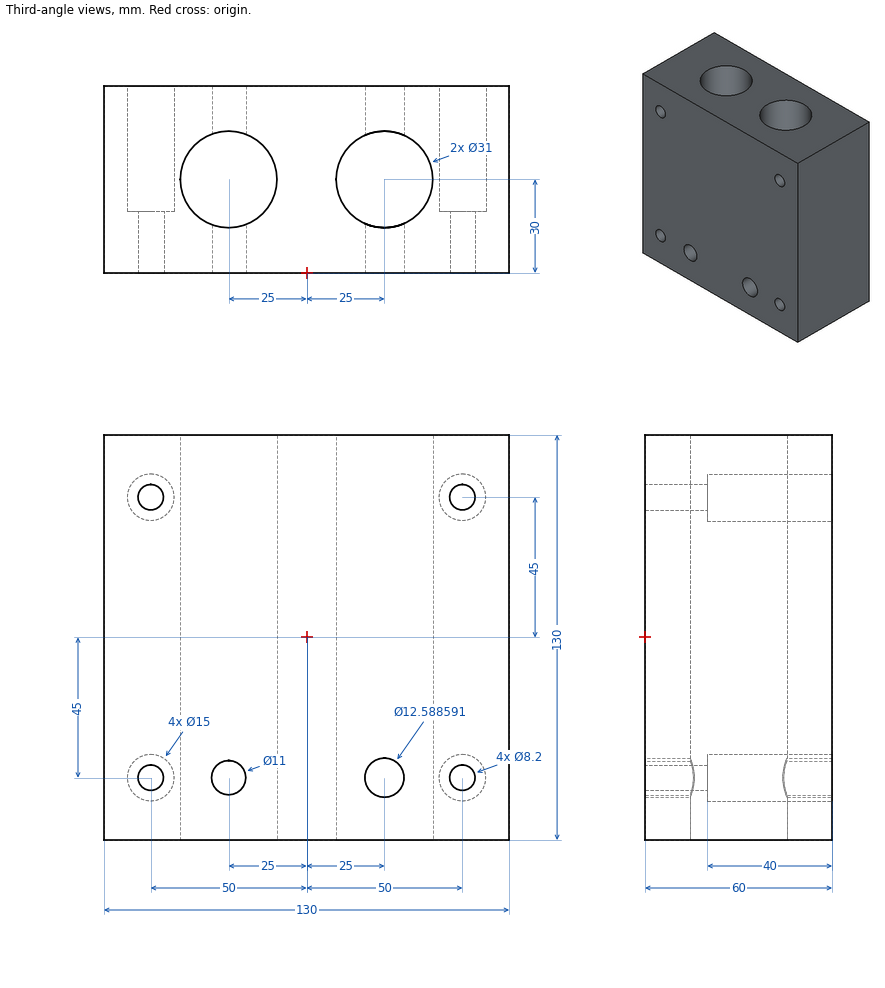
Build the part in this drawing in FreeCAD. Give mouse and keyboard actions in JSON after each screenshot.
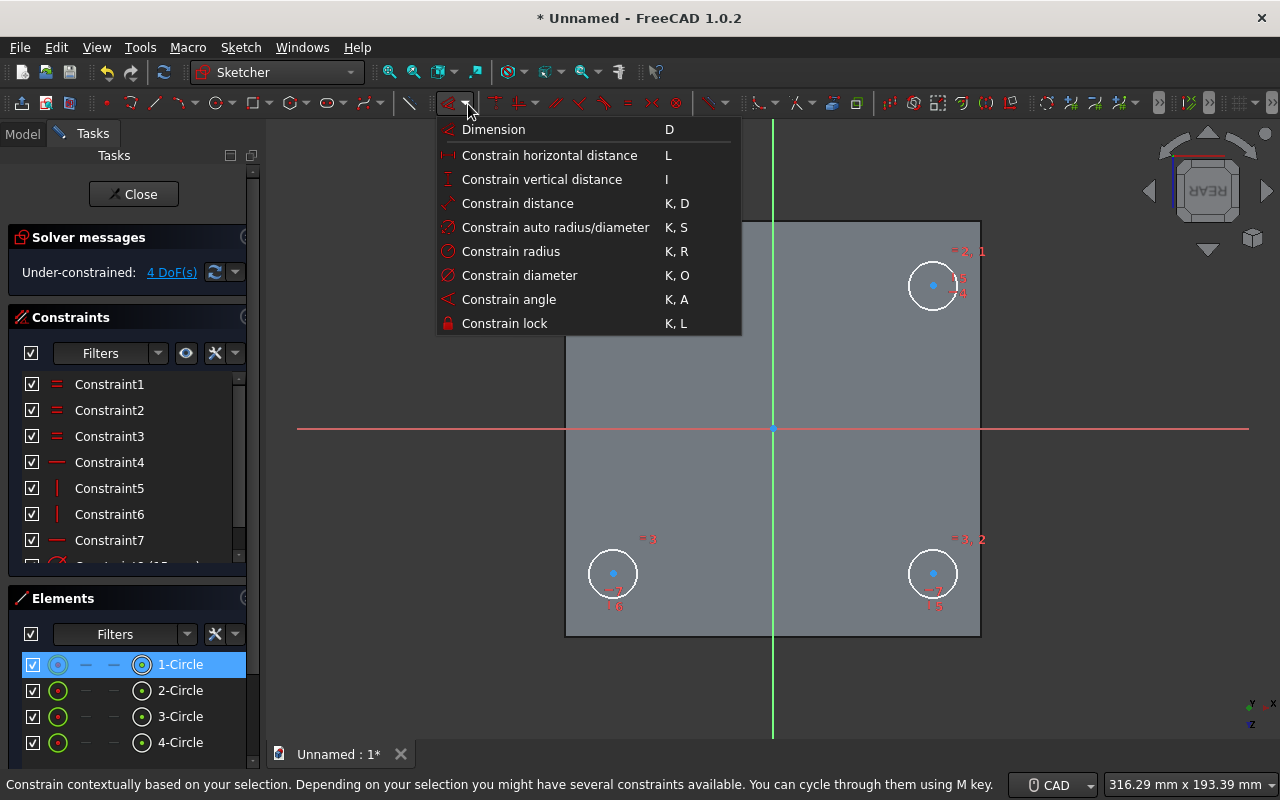
{"action": "left_click", "coordinate": [589, 155]}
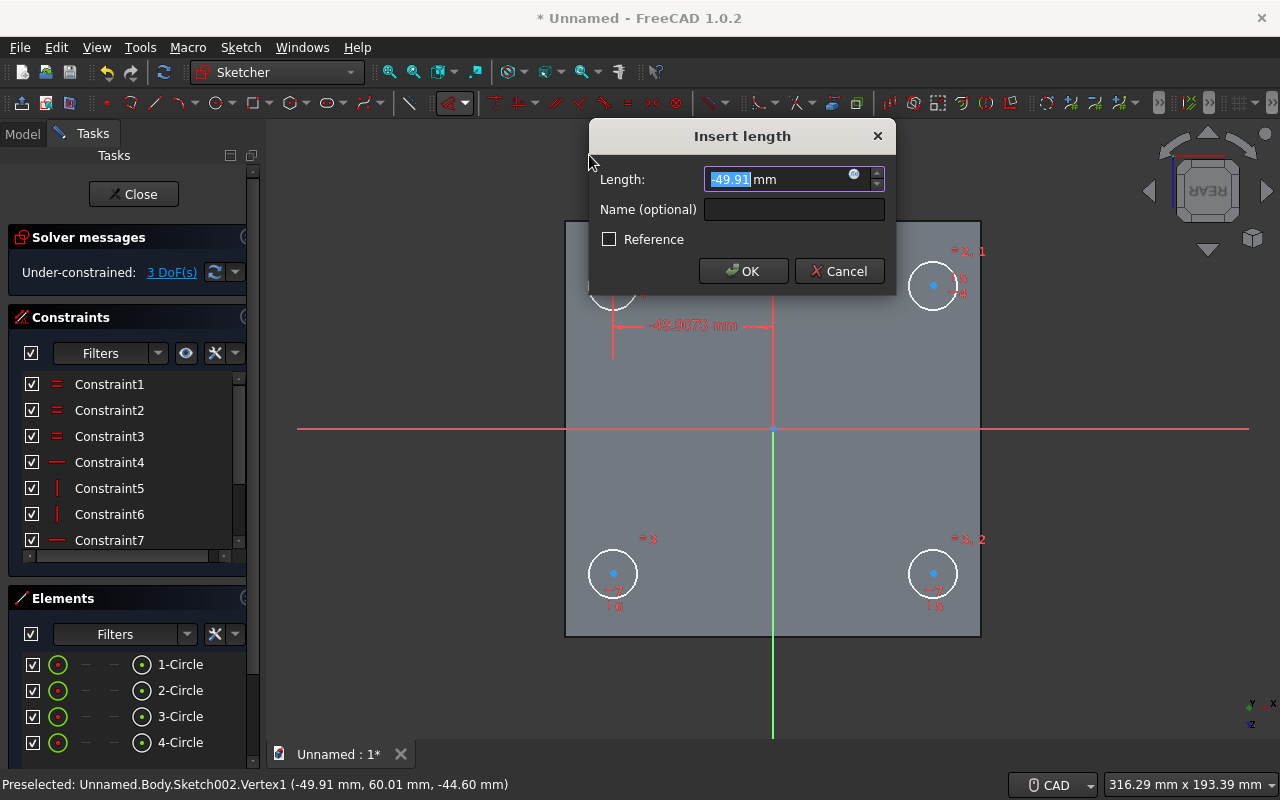
{"action": "type", "text": "-50"}
{"action": "key", "text": "Return"}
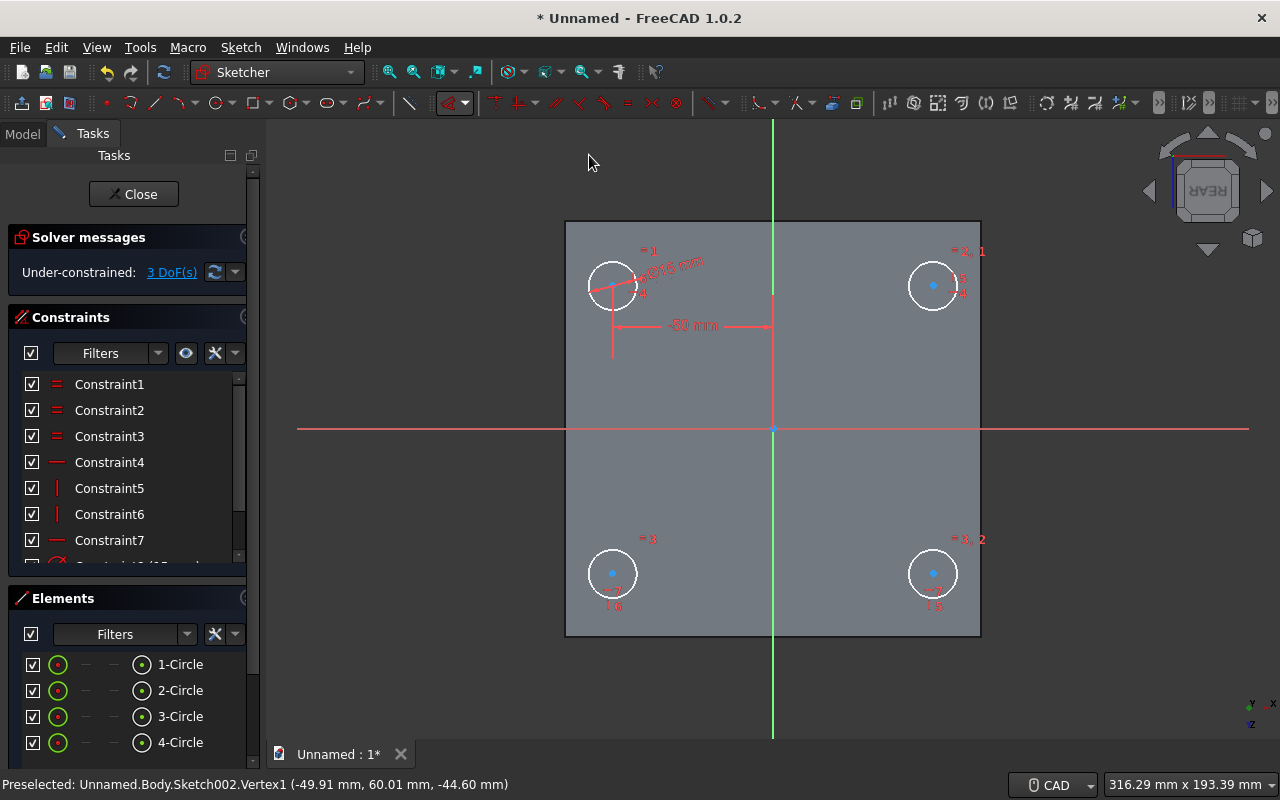
{"action": "left_click", "coordinate": [613, 286]}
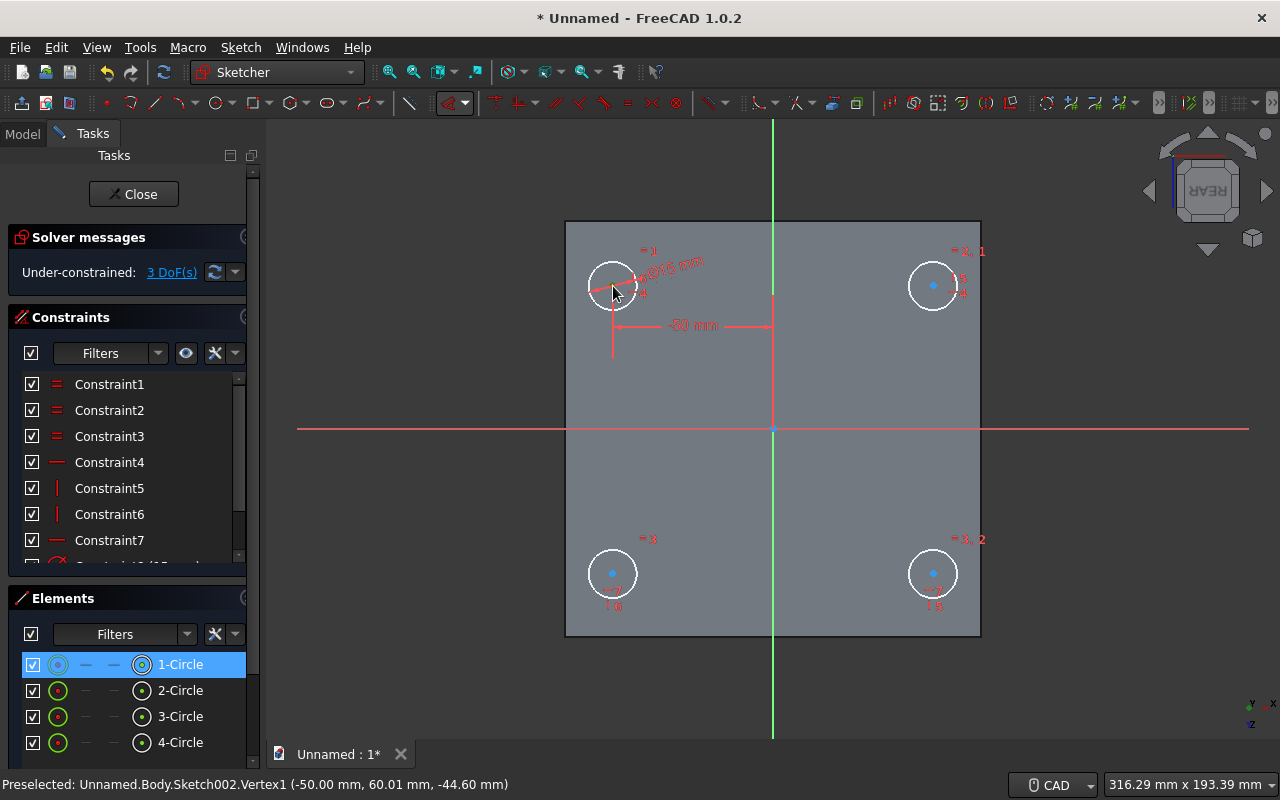
{"action": "key", "text": "i"}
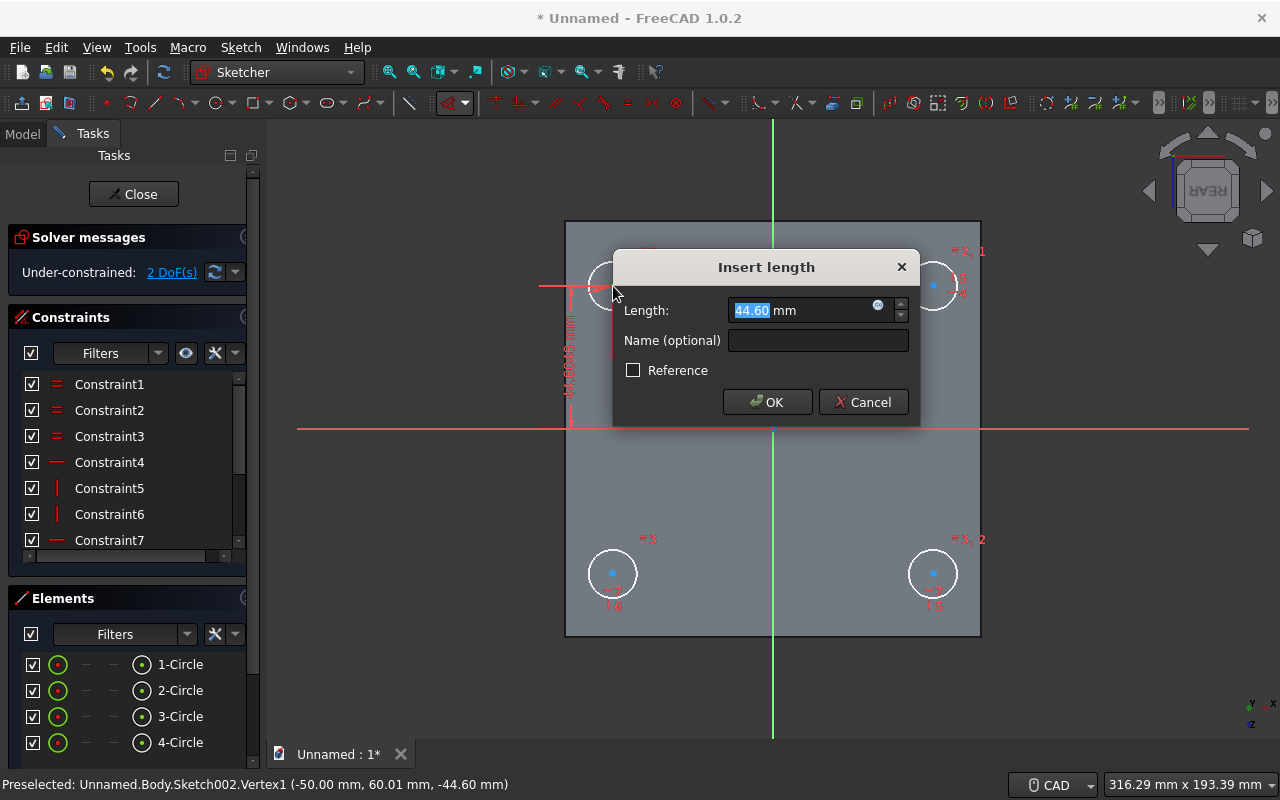
{"action": "type", "text": "45"}
{"action": "key", "text": "Return"}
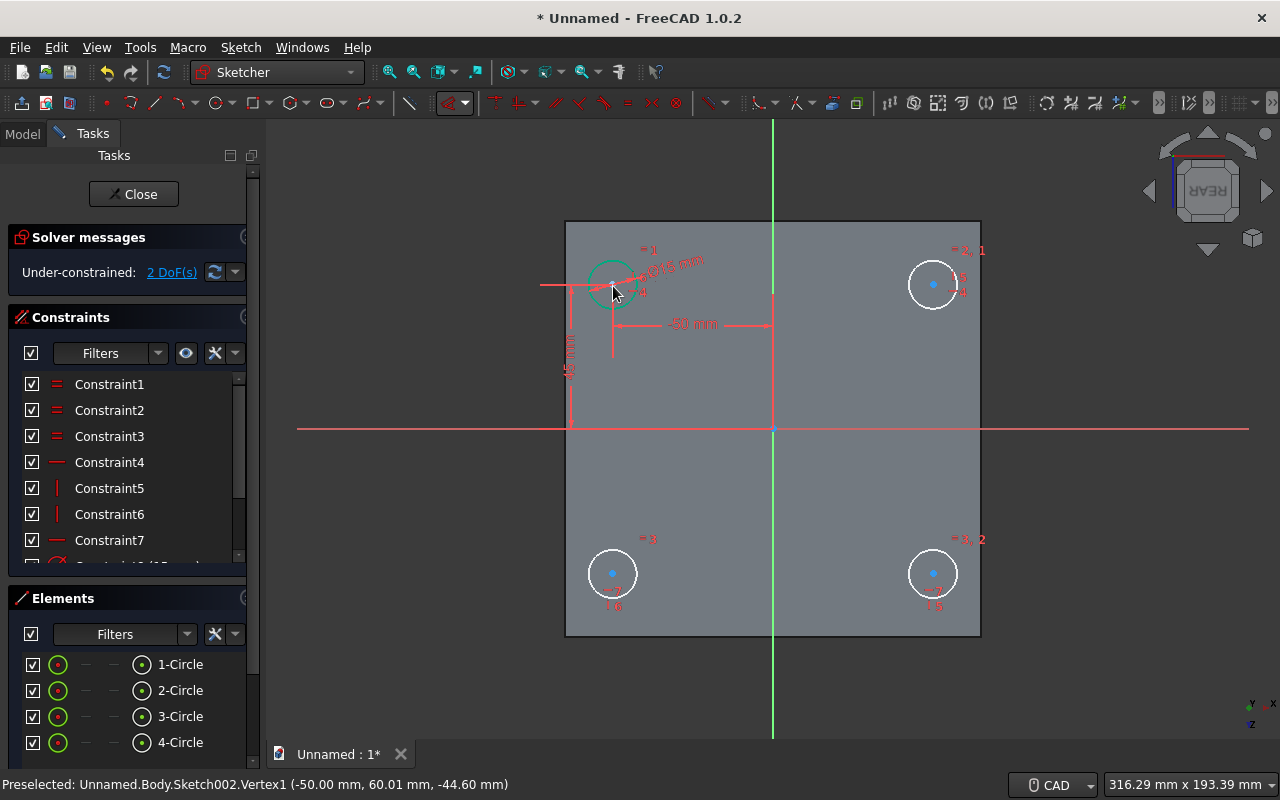
{"action": "left_click", "coordinate": [933, 285]}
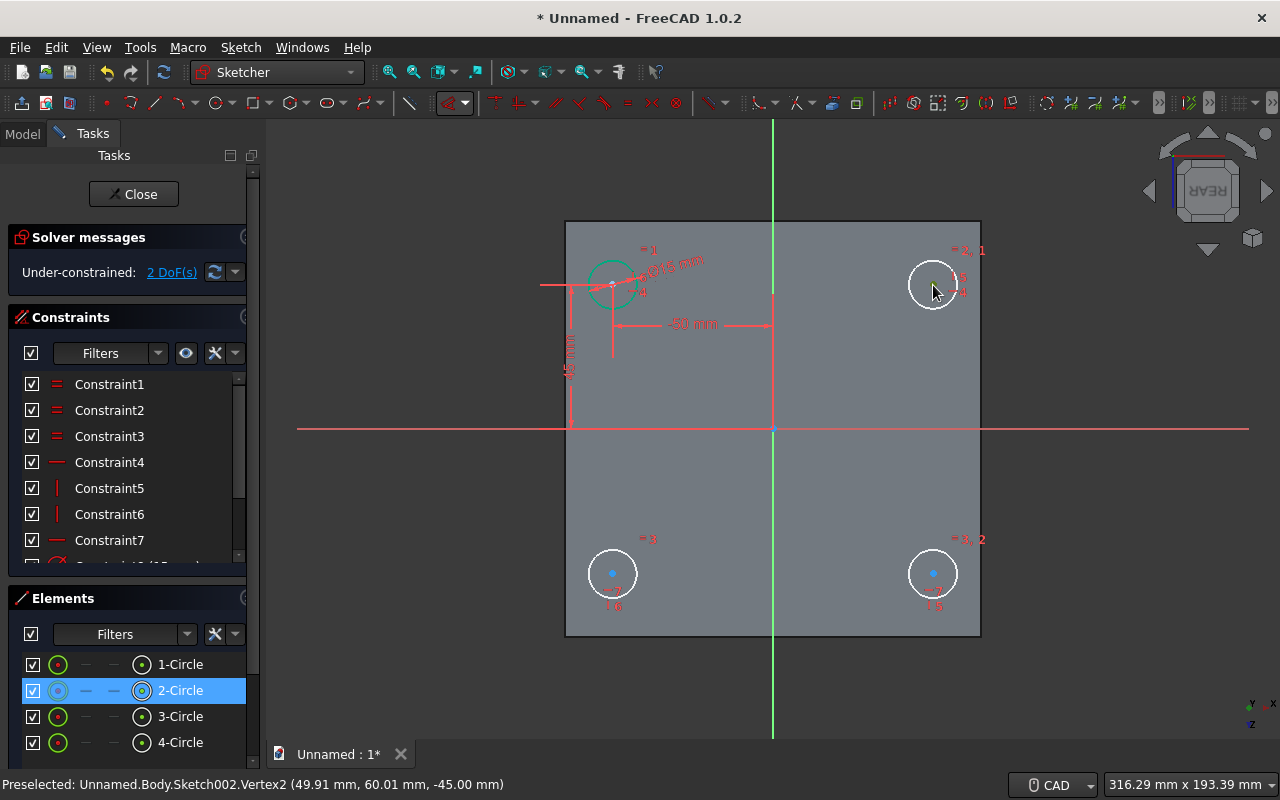
{"action": "key", "text": "l"}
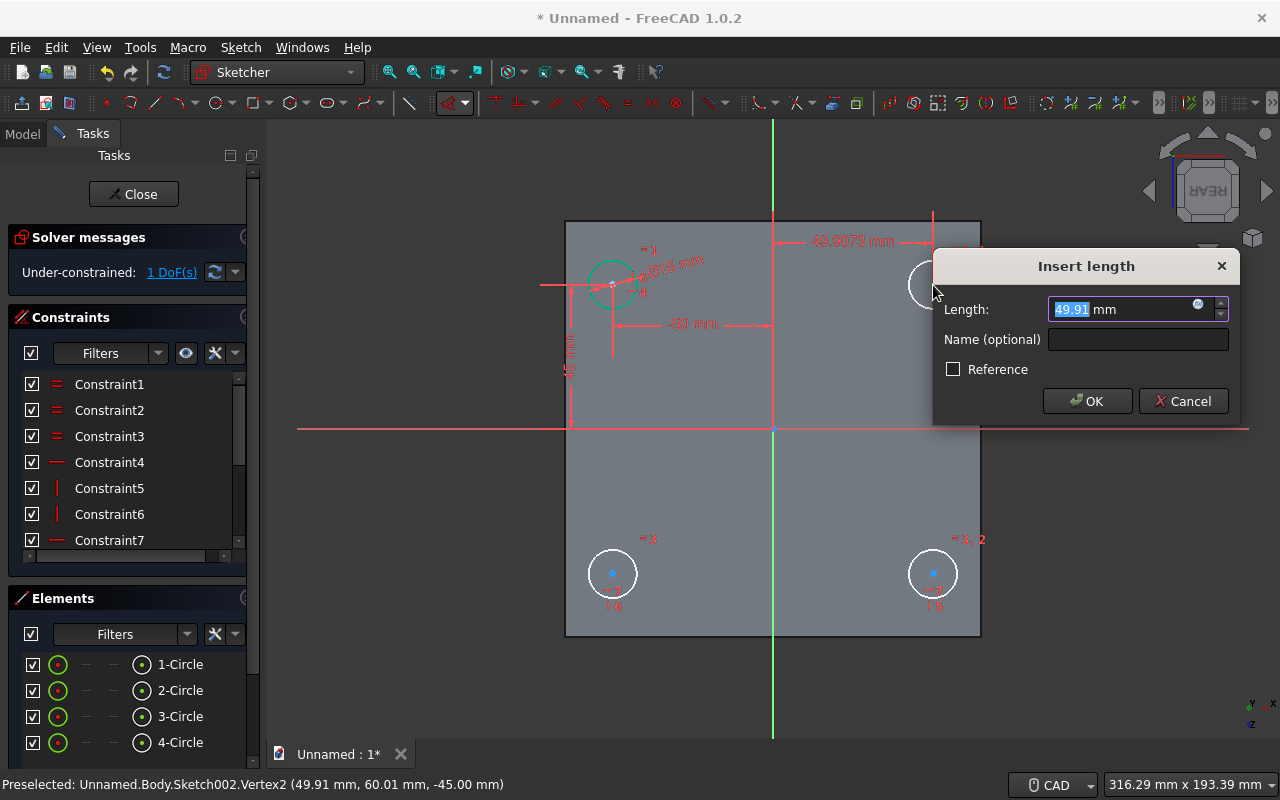
{"action": "type", "text": "50"}
{"action": "key", "text": "Return"}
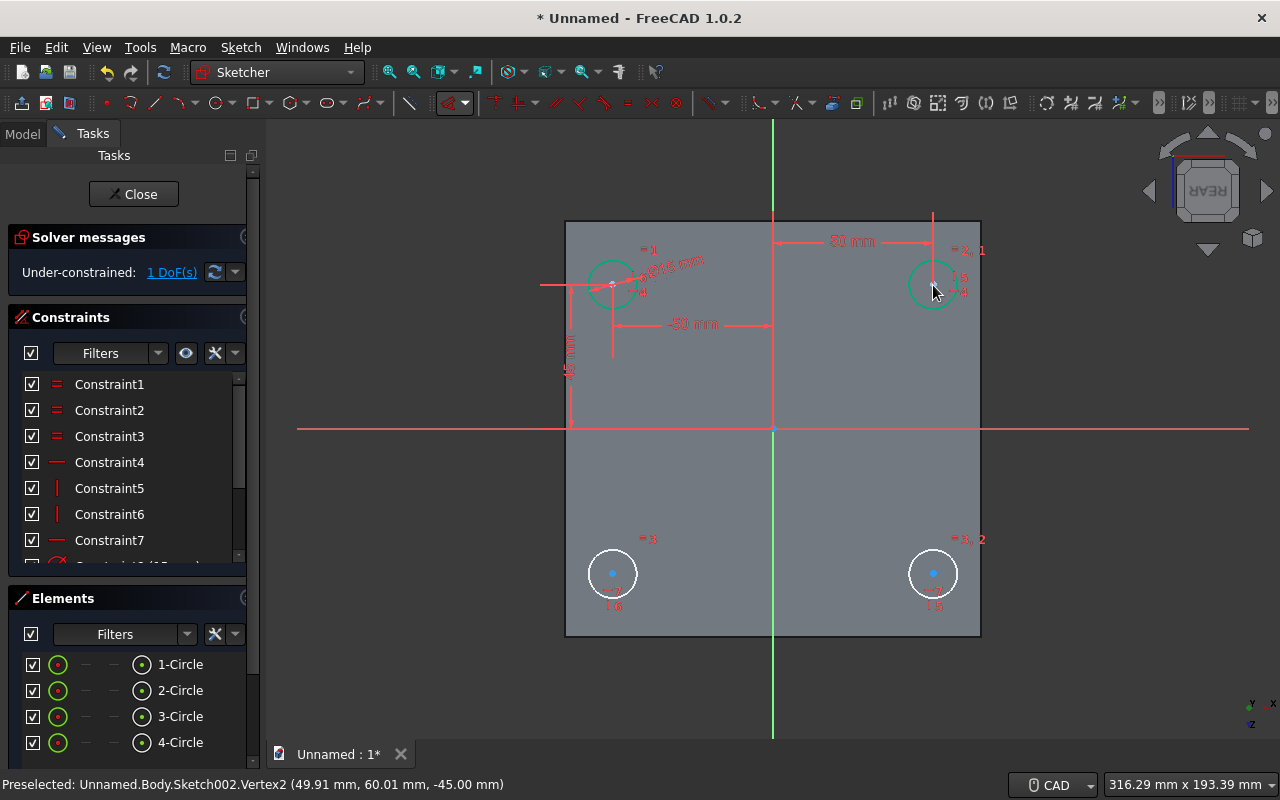
{"action": "left_click", "coordinate": [933, 574]}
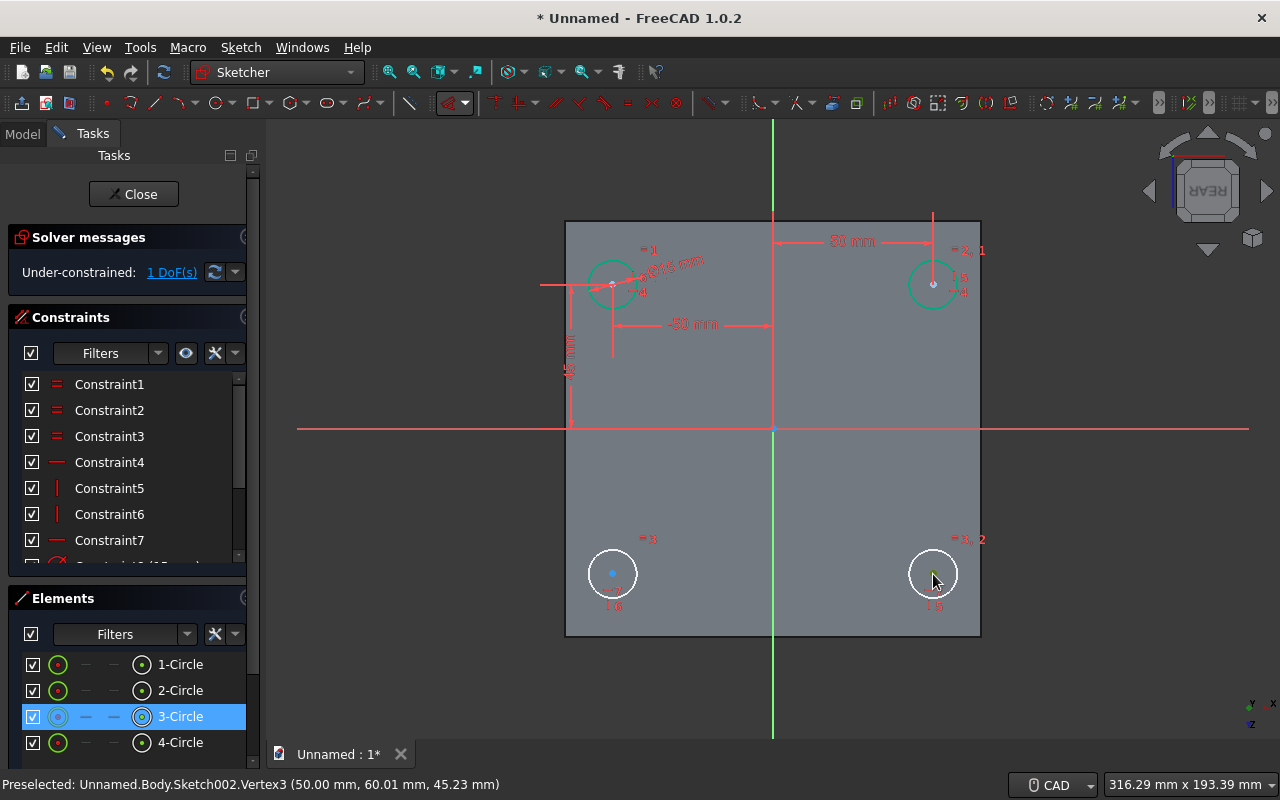
{"action": "key", "text": "i"}